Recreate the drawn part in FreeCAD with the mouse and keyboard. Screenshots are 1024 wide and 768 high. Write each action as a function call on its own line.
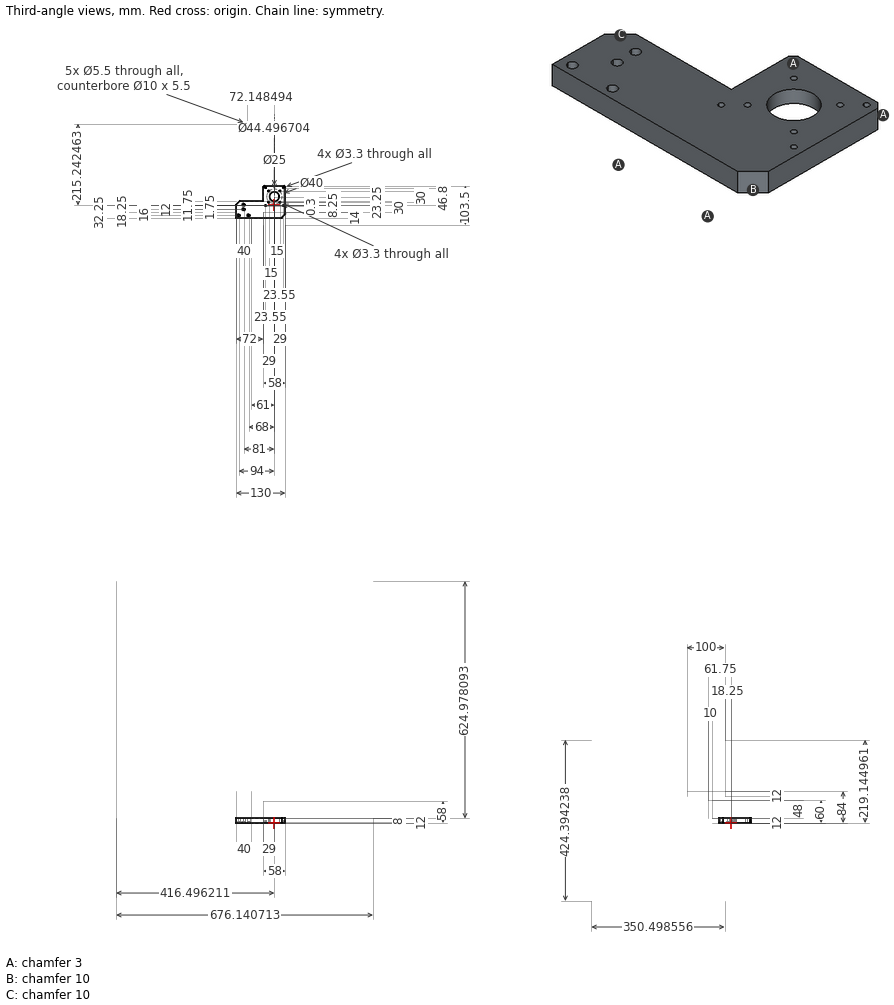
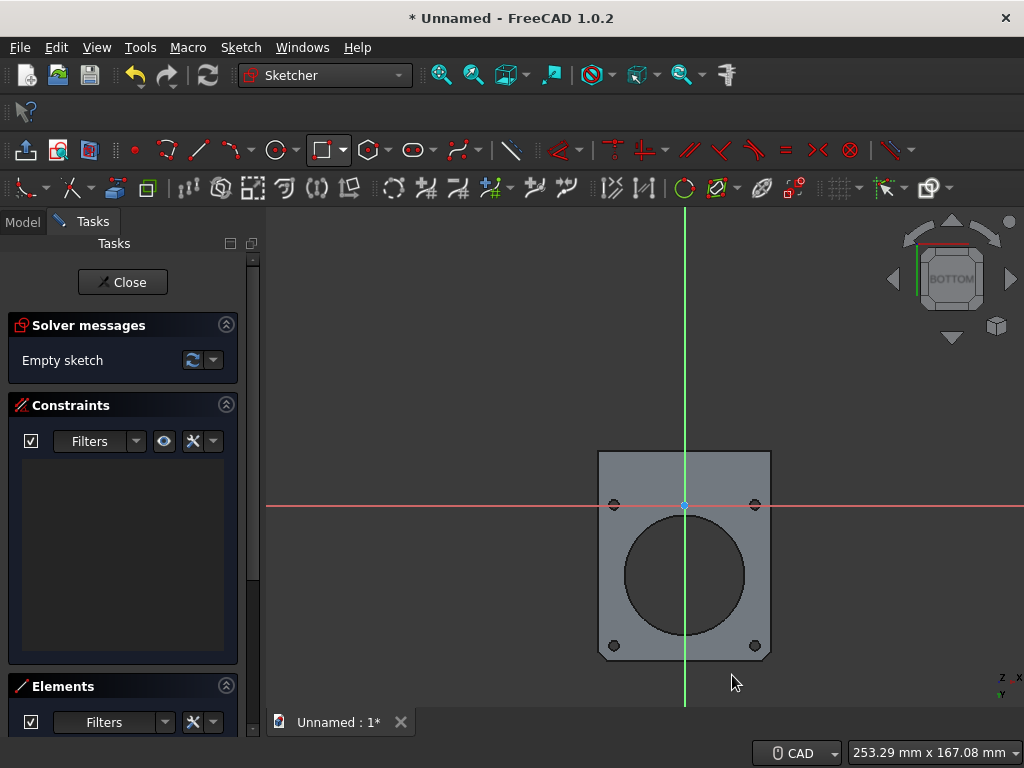
click(322, 150)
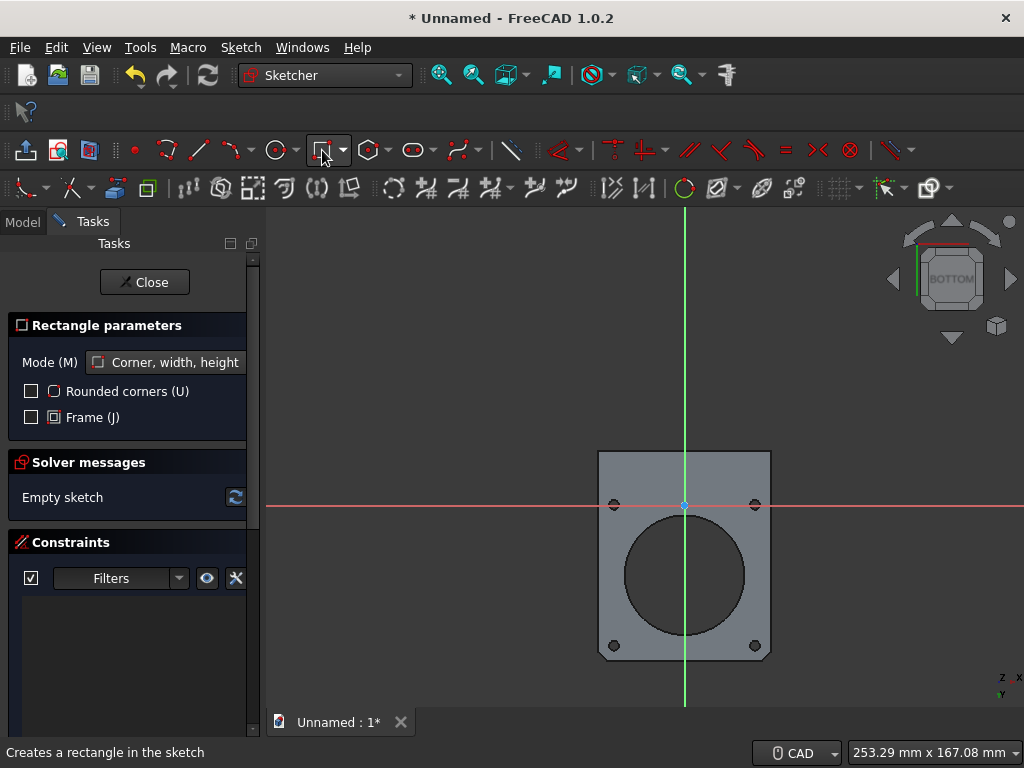
click(382, 409)
move(771, 451)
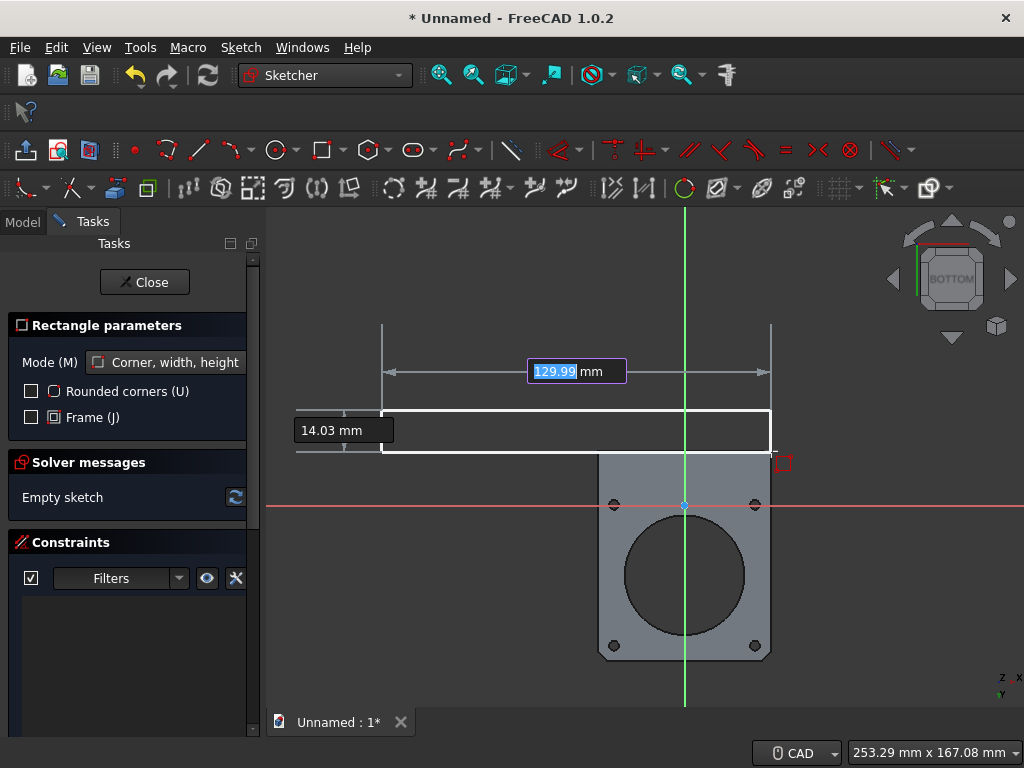
text(130)
key(Tab)
text(14)
key(Return)
key(Escape)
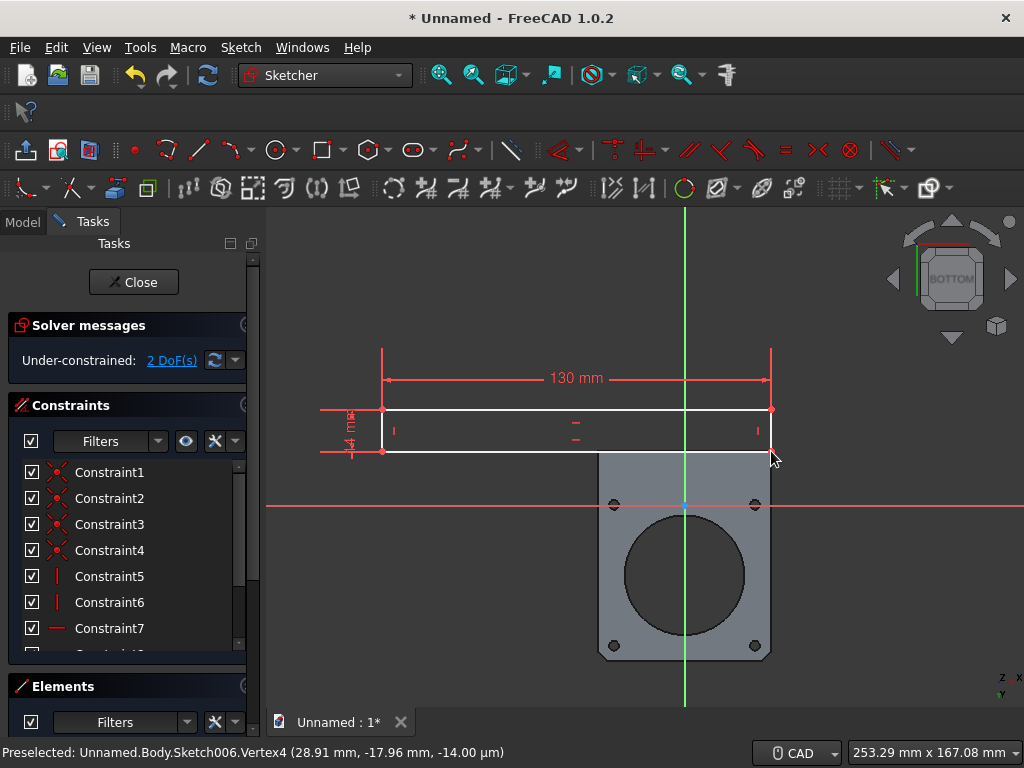
key(d)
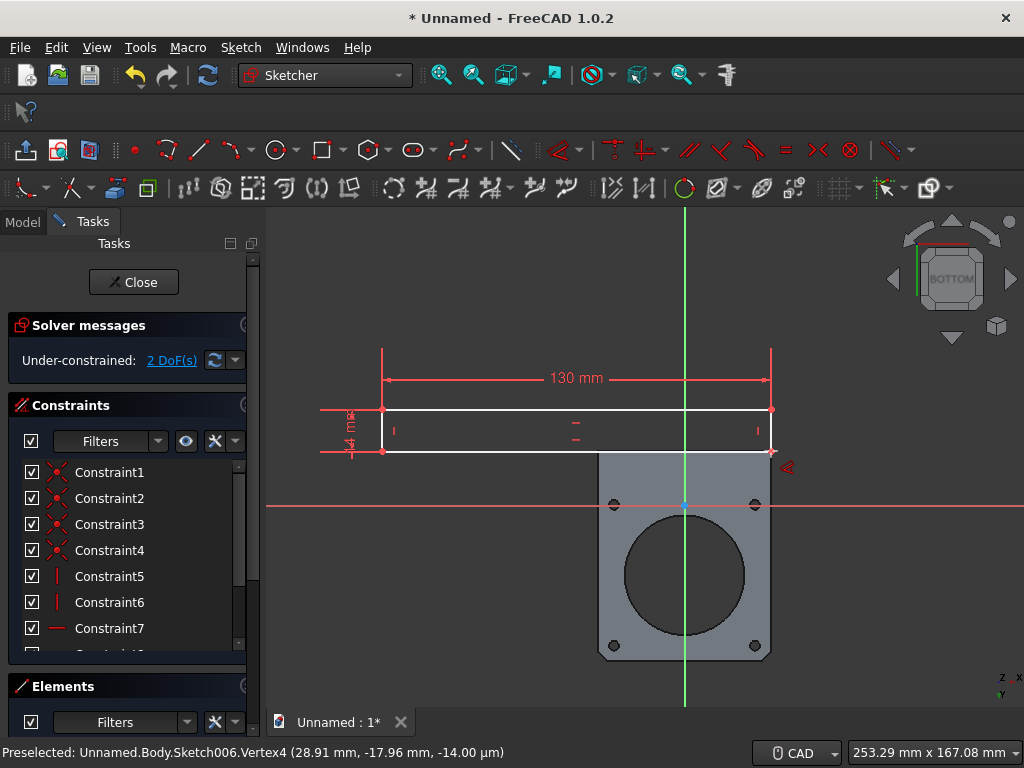
click(771, 452)
click(728, 540)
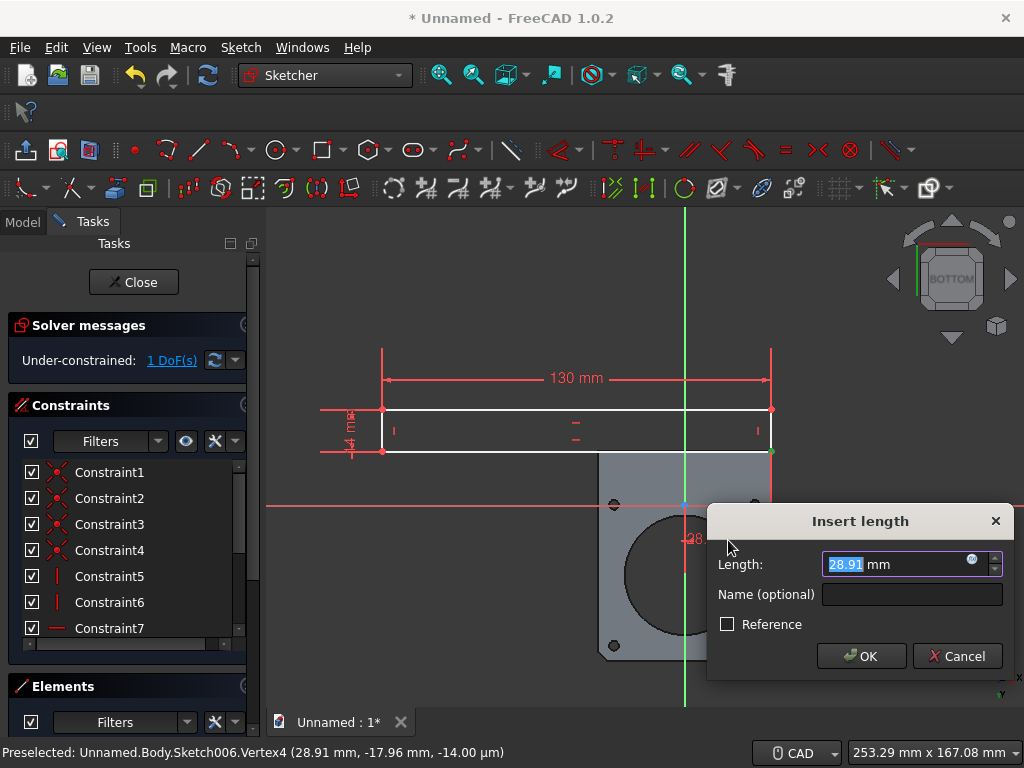
text(29)
key(Return)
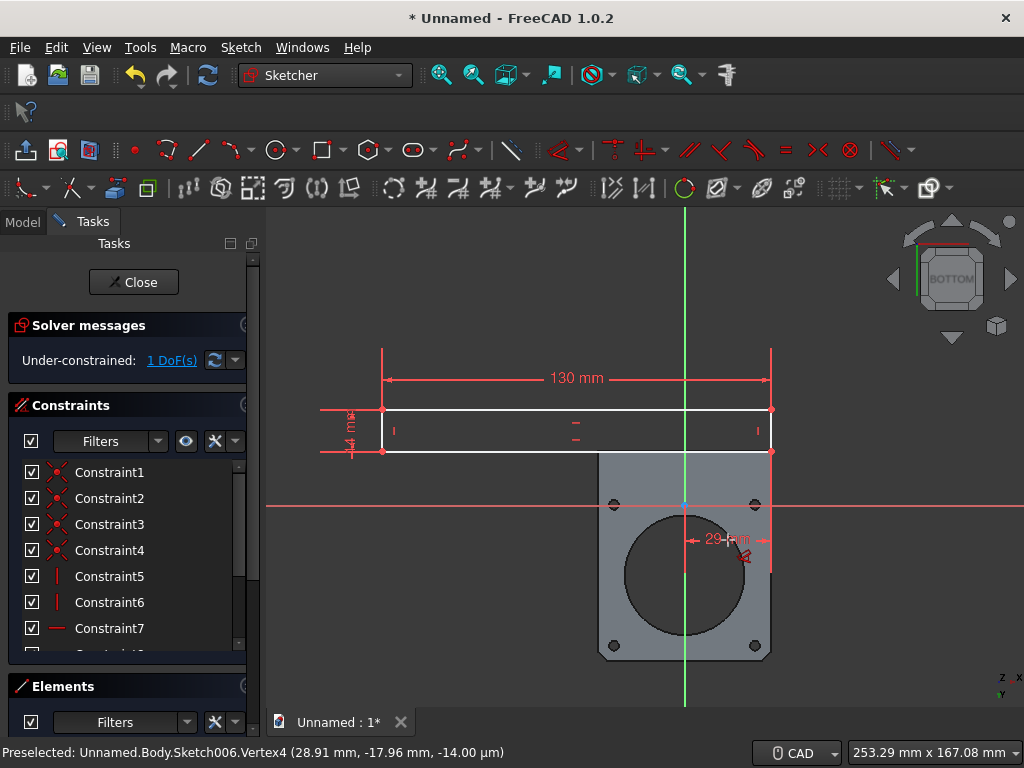
click(382, 410)
click(348, 458)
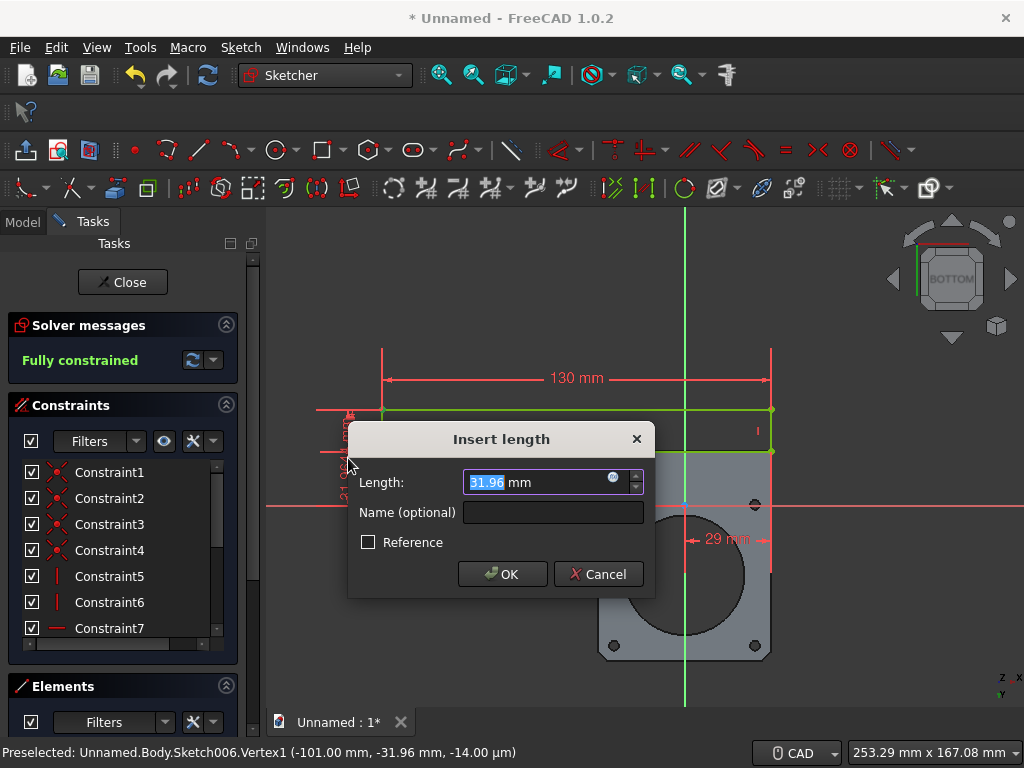
text(32.25)
key(Return)
key(Escape)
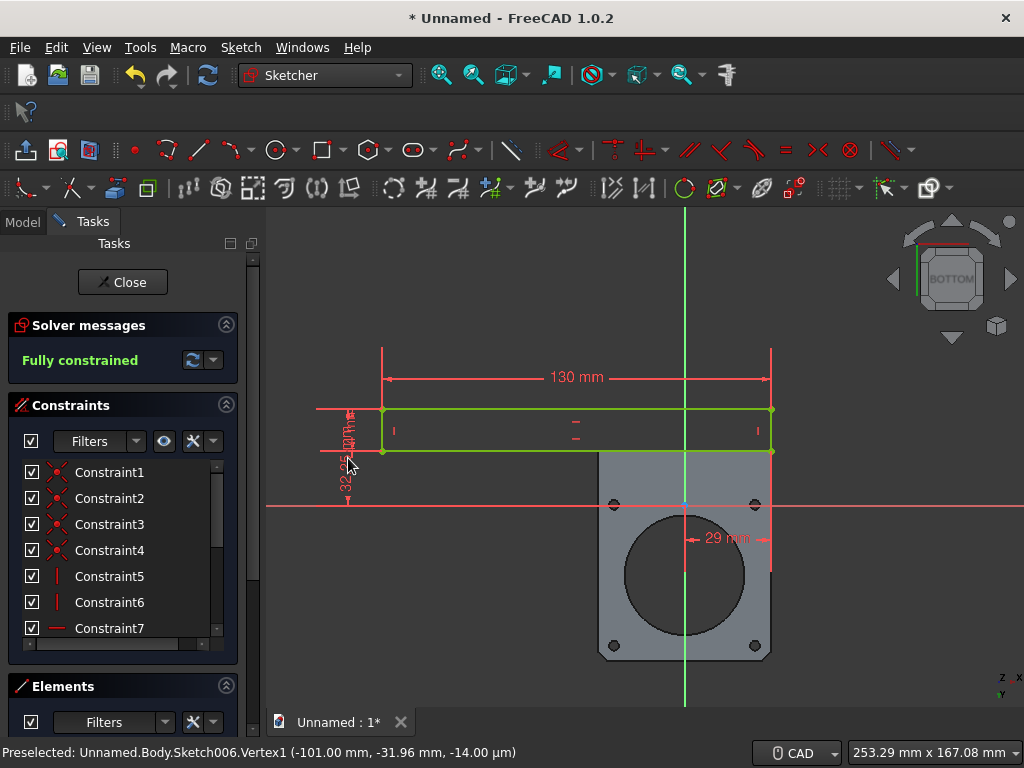
click(123, 282)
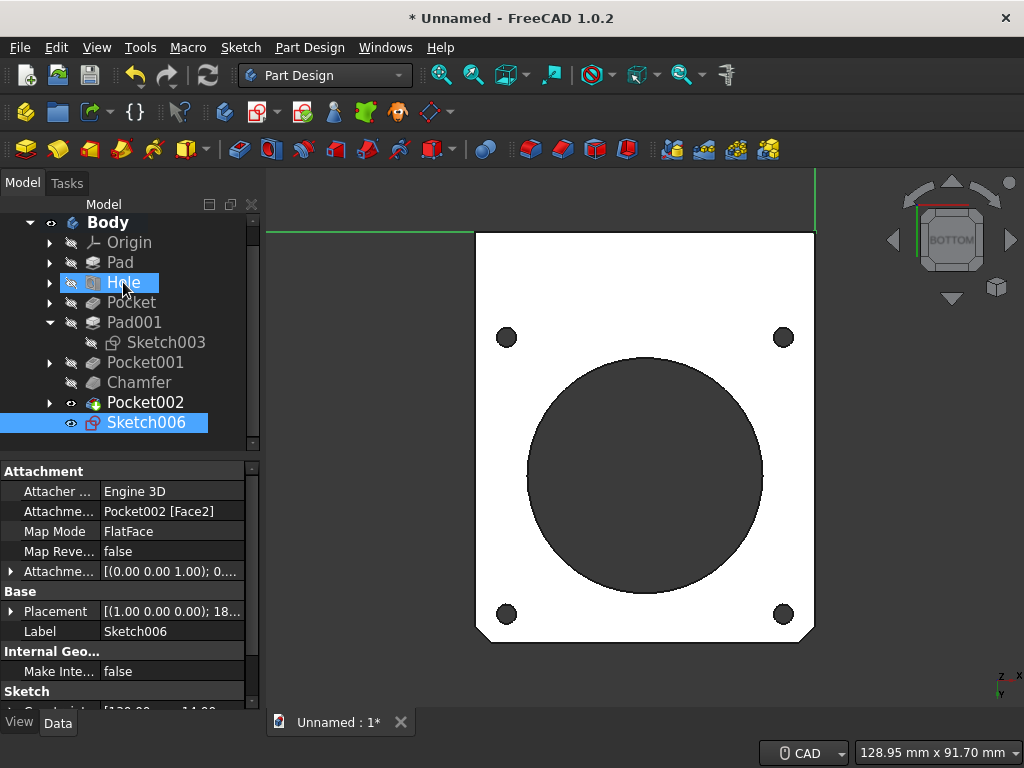
click(26, 150)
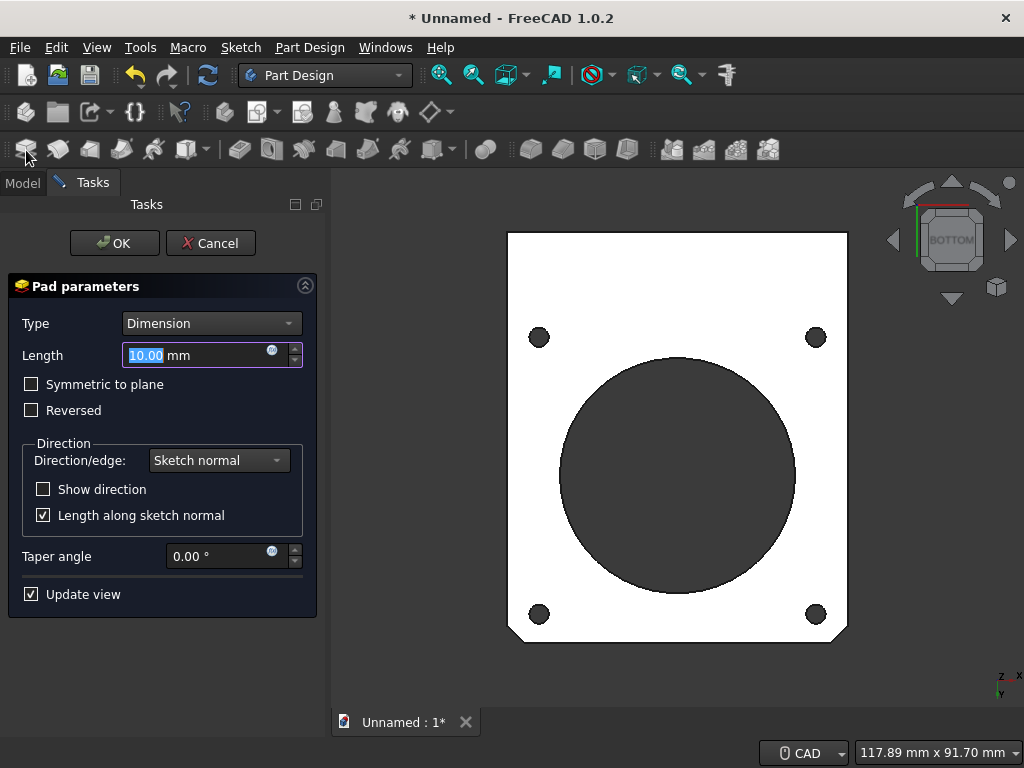
text(12)
key(Tab)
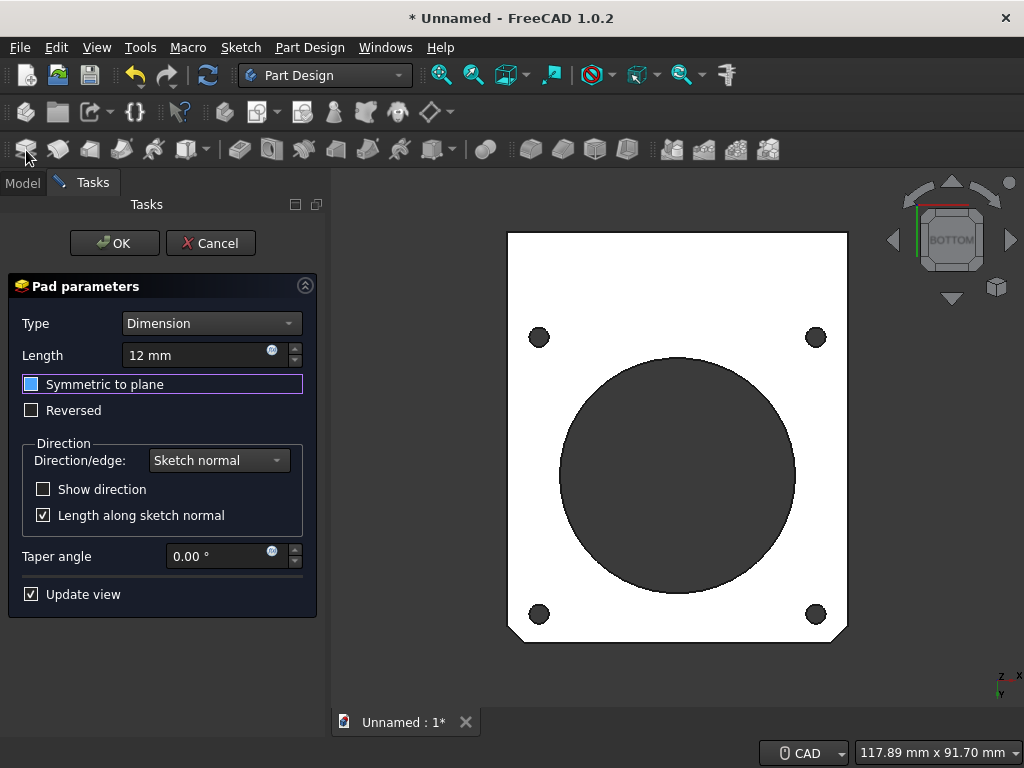
click(30, 410)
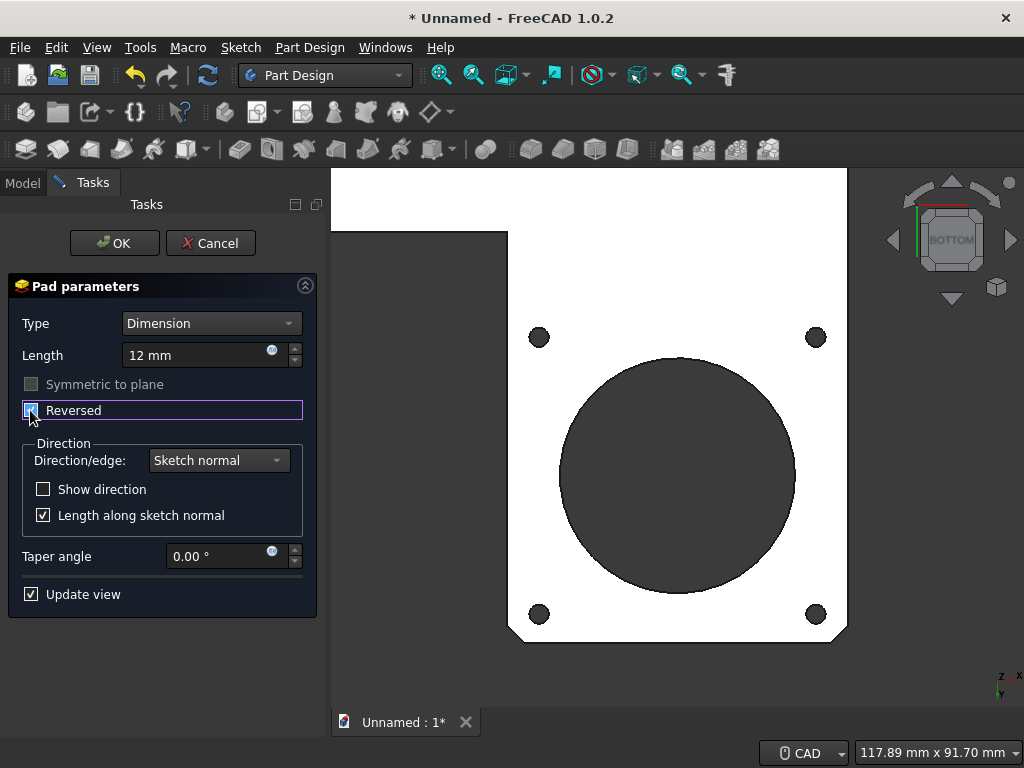
click(115, 243)